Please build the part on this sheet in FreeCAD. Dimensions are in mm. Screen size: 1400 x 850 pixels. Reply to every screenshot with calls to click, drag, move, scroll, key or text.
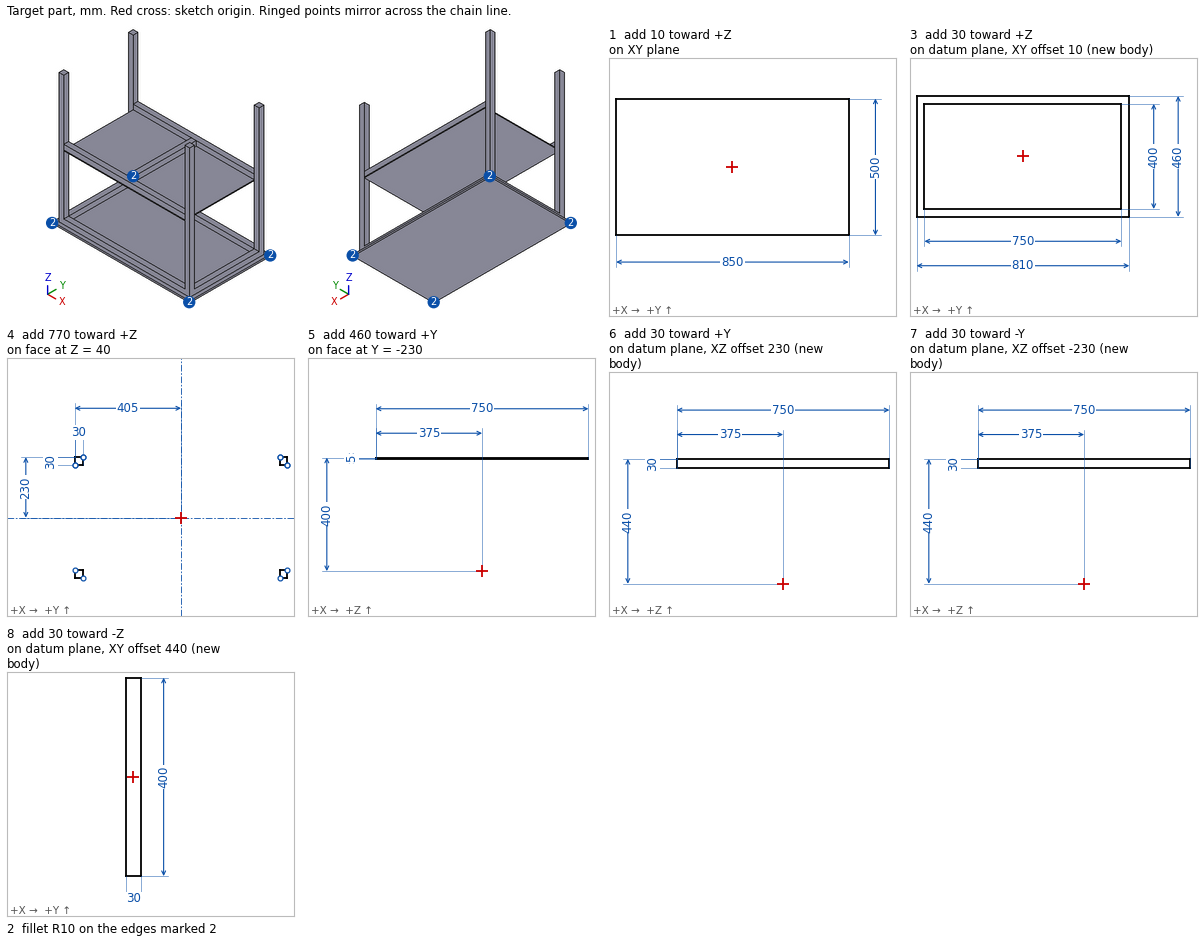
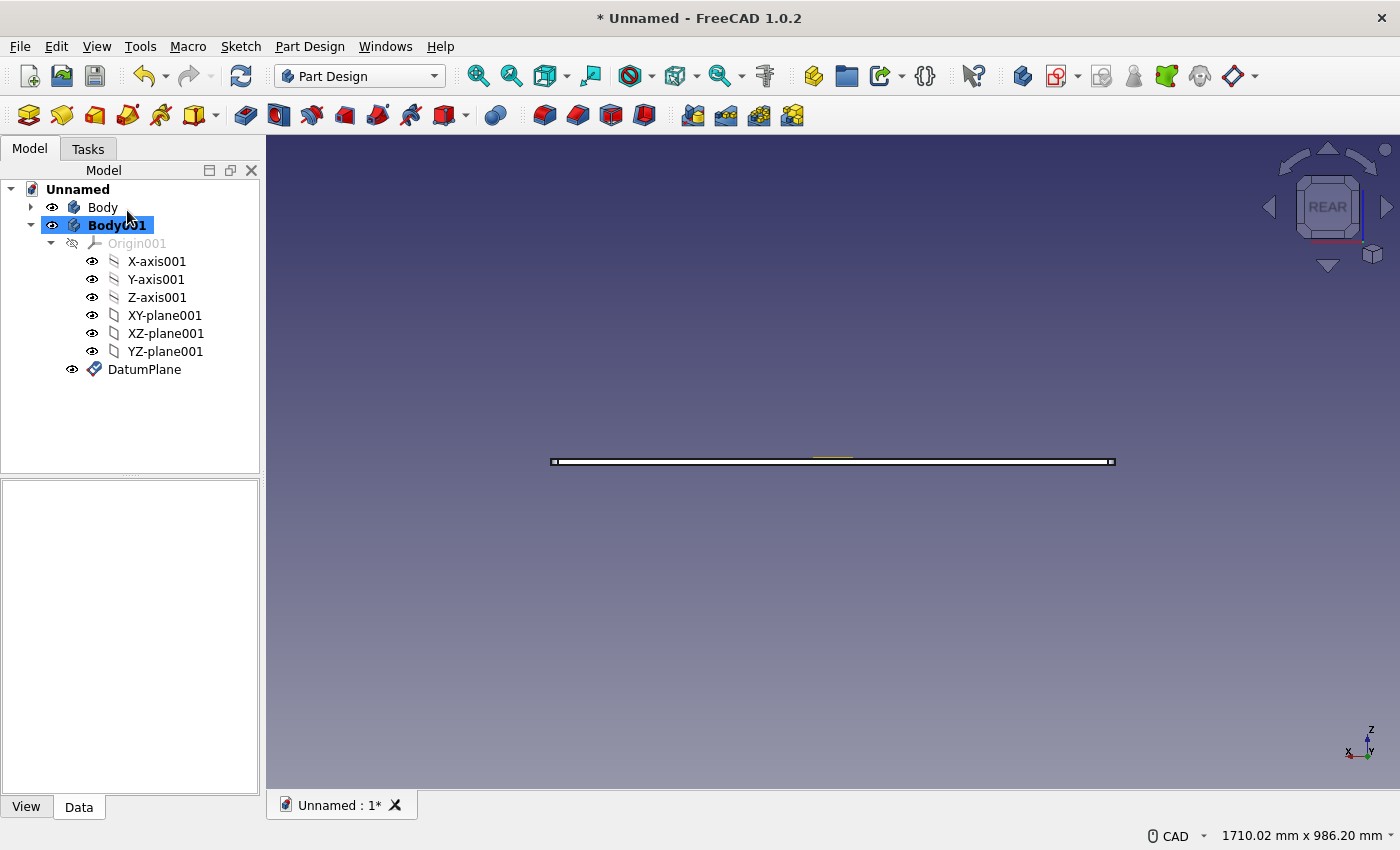
click(117, 369)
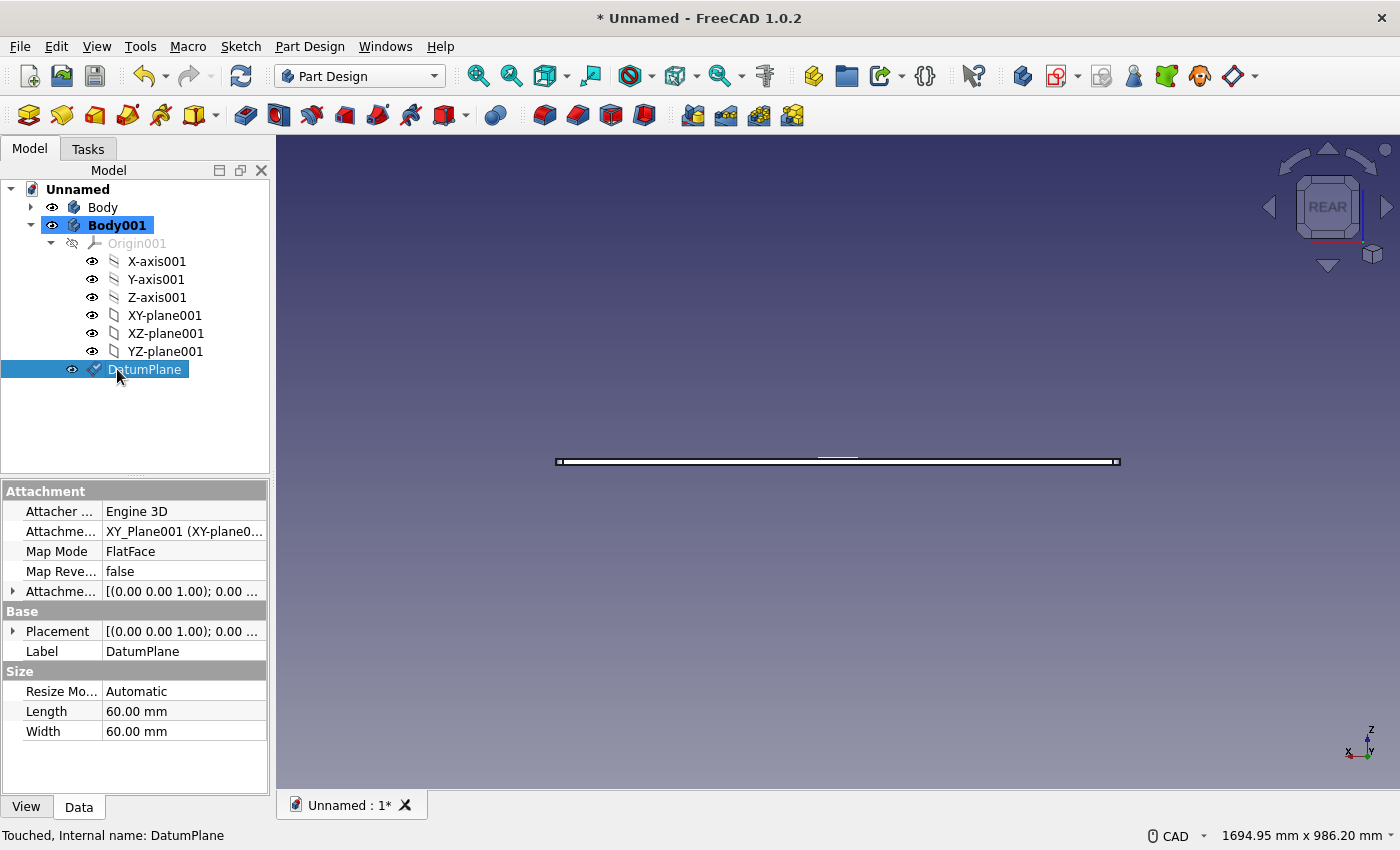
click(1056, 76)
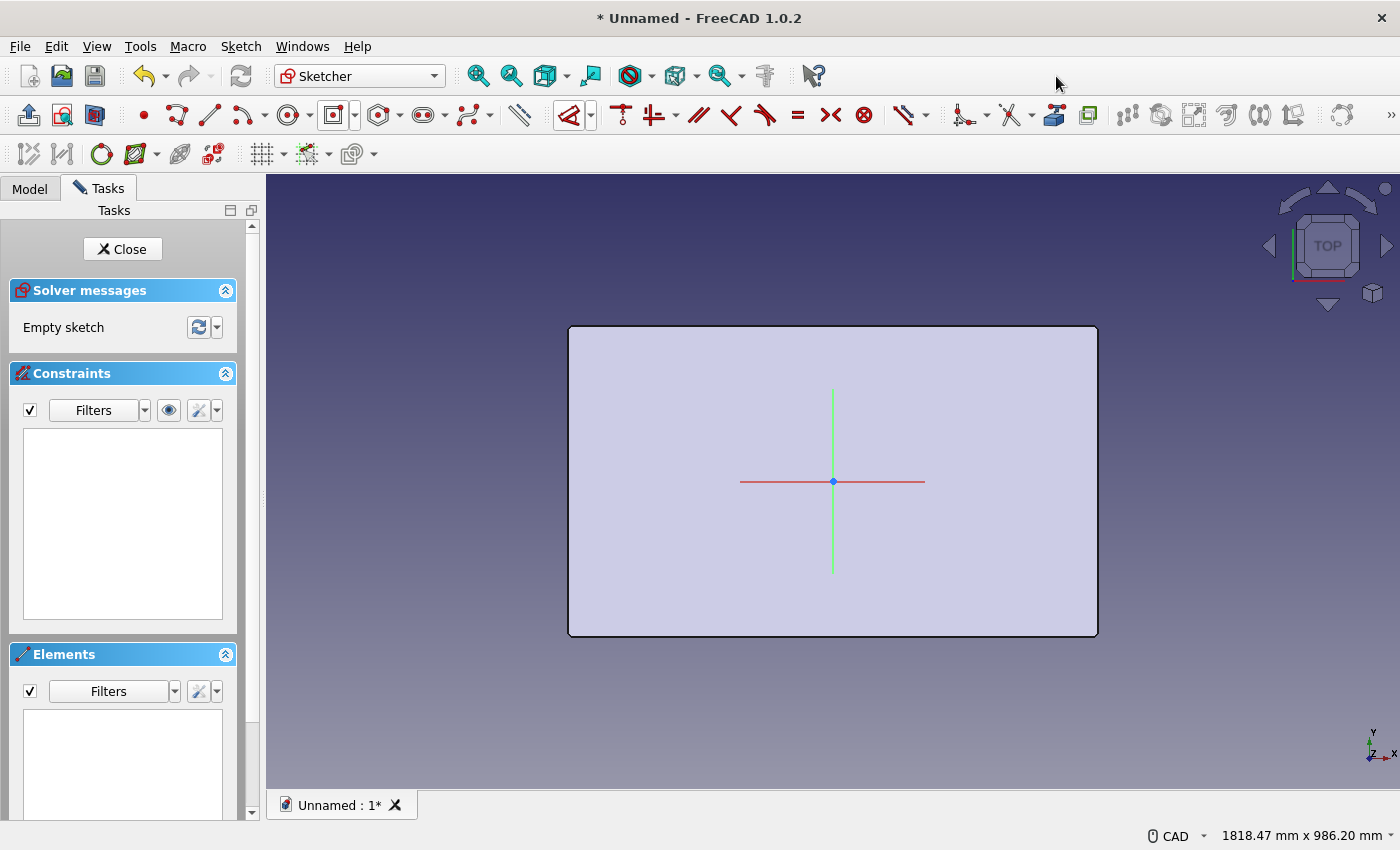
click(332, 116)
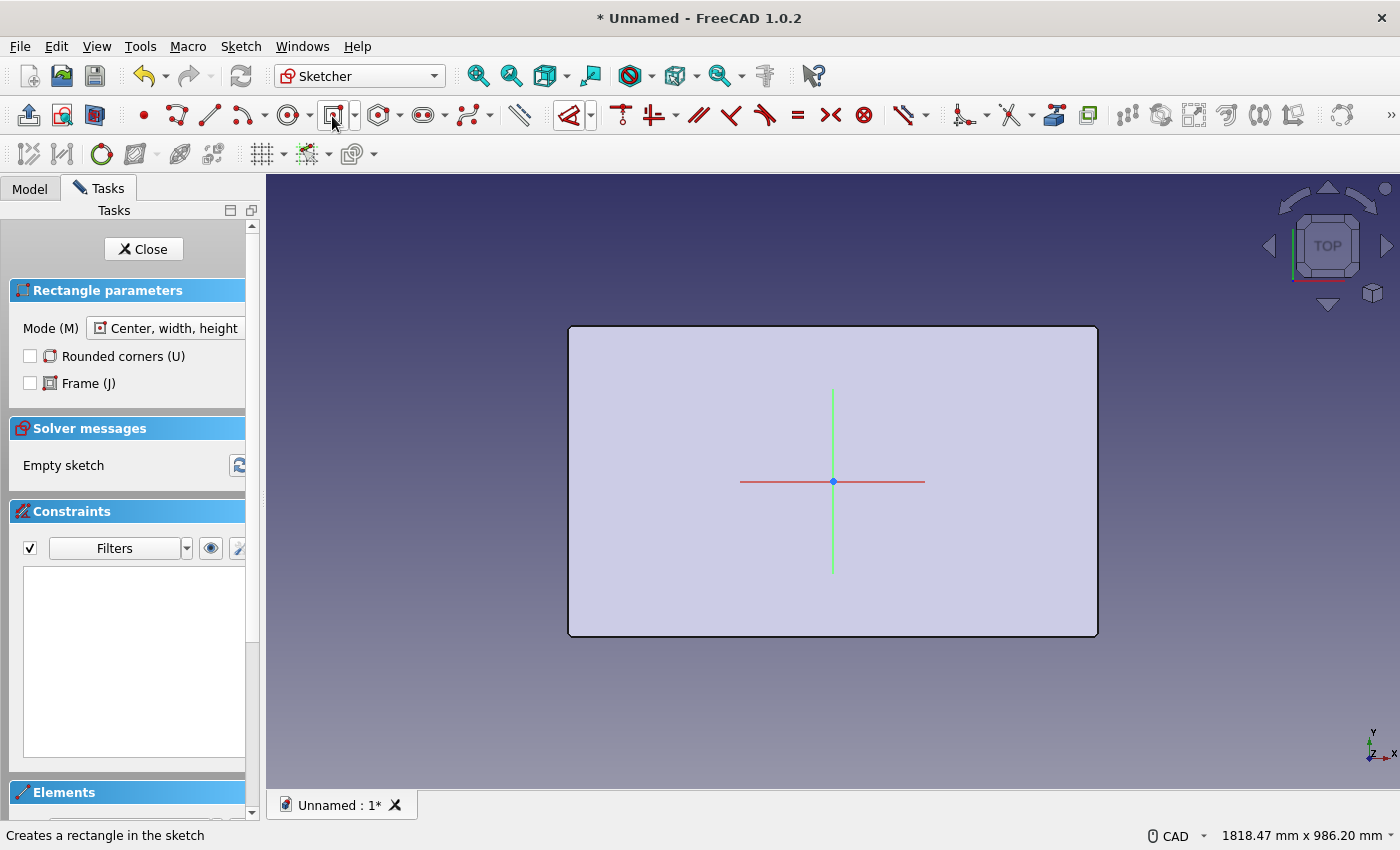
click(833, 482)
click(1086, 338)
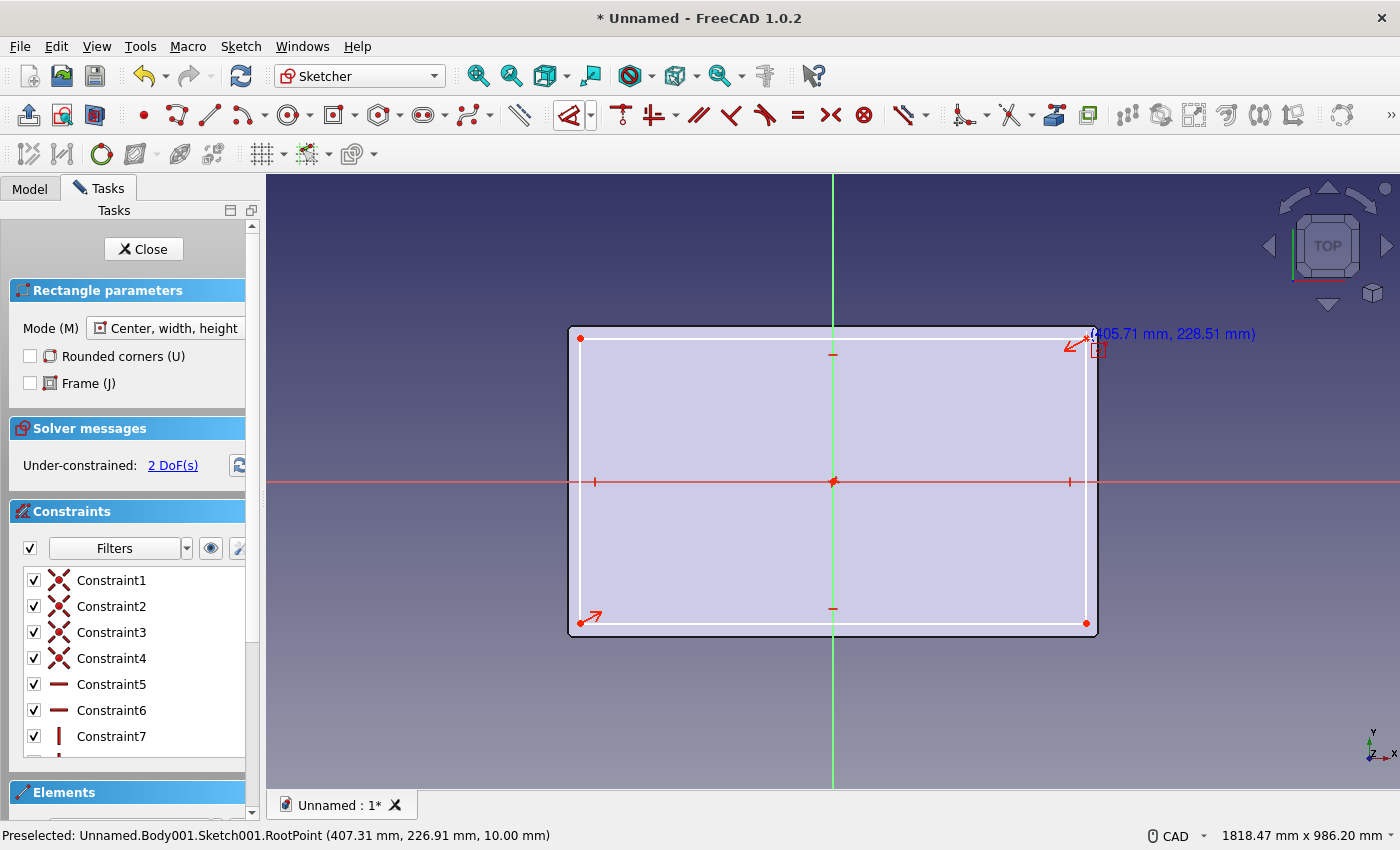
click(833, 482)
click(1067, 357)
key(Escape)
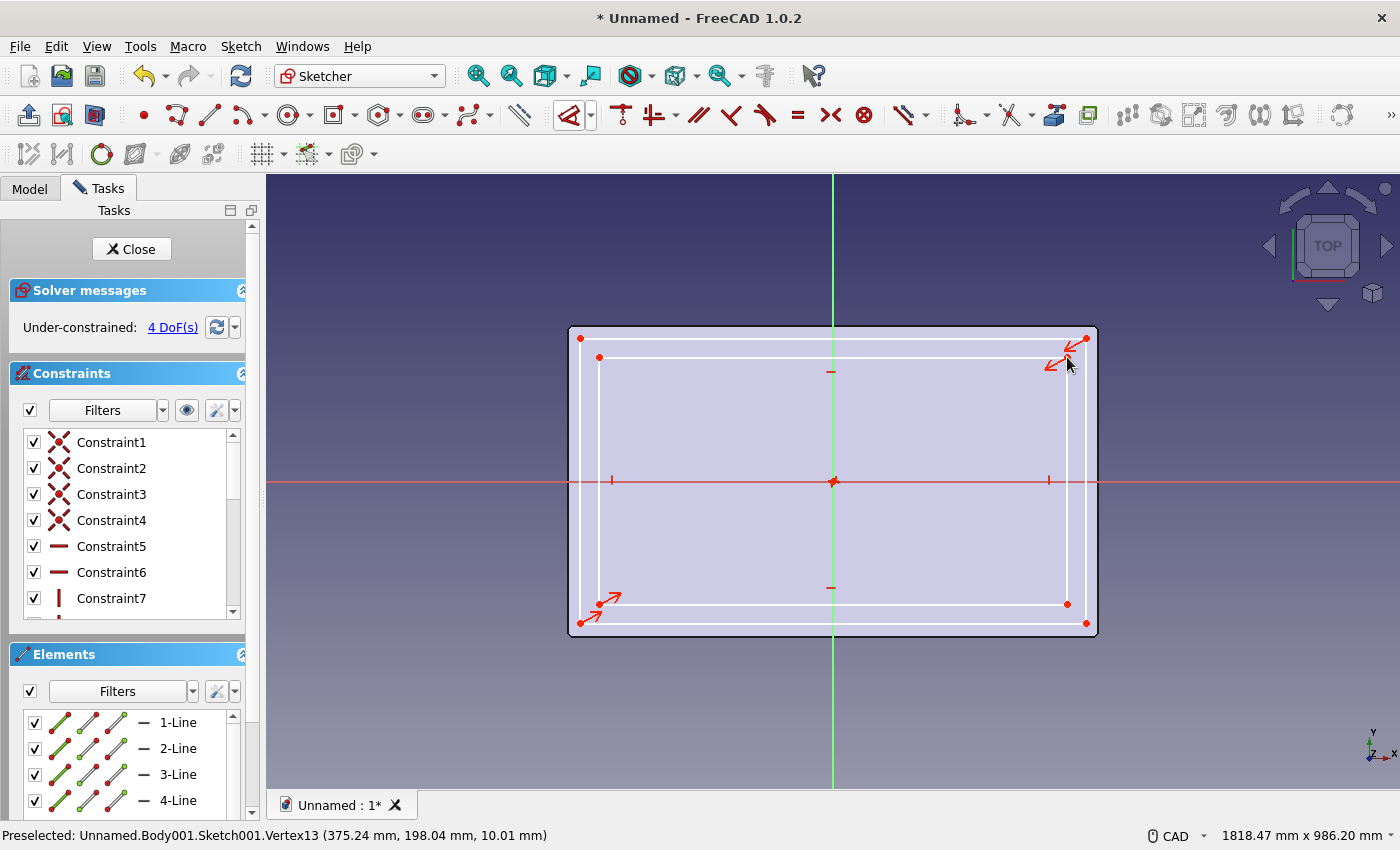
click(732, 624)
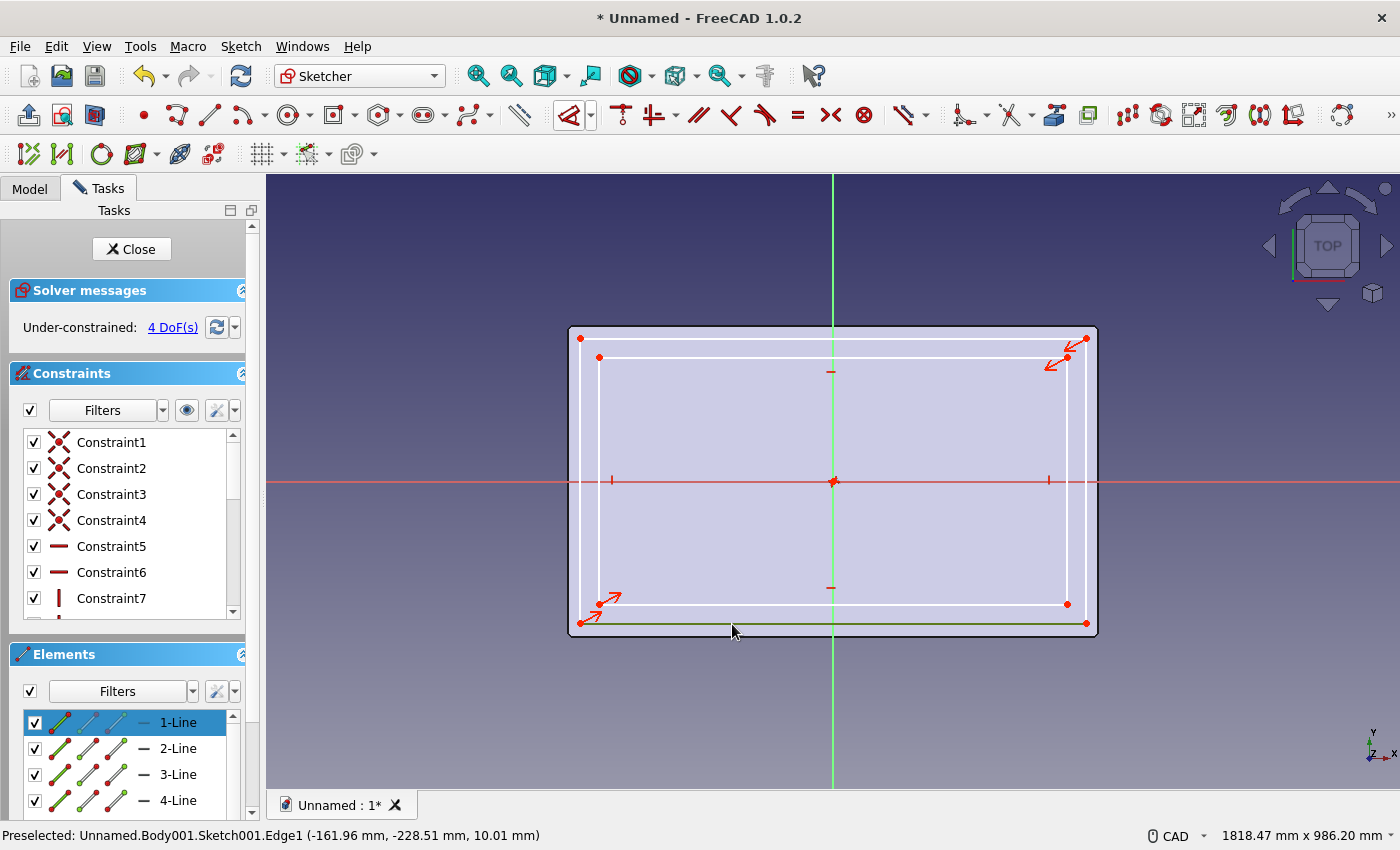
click(590, 116)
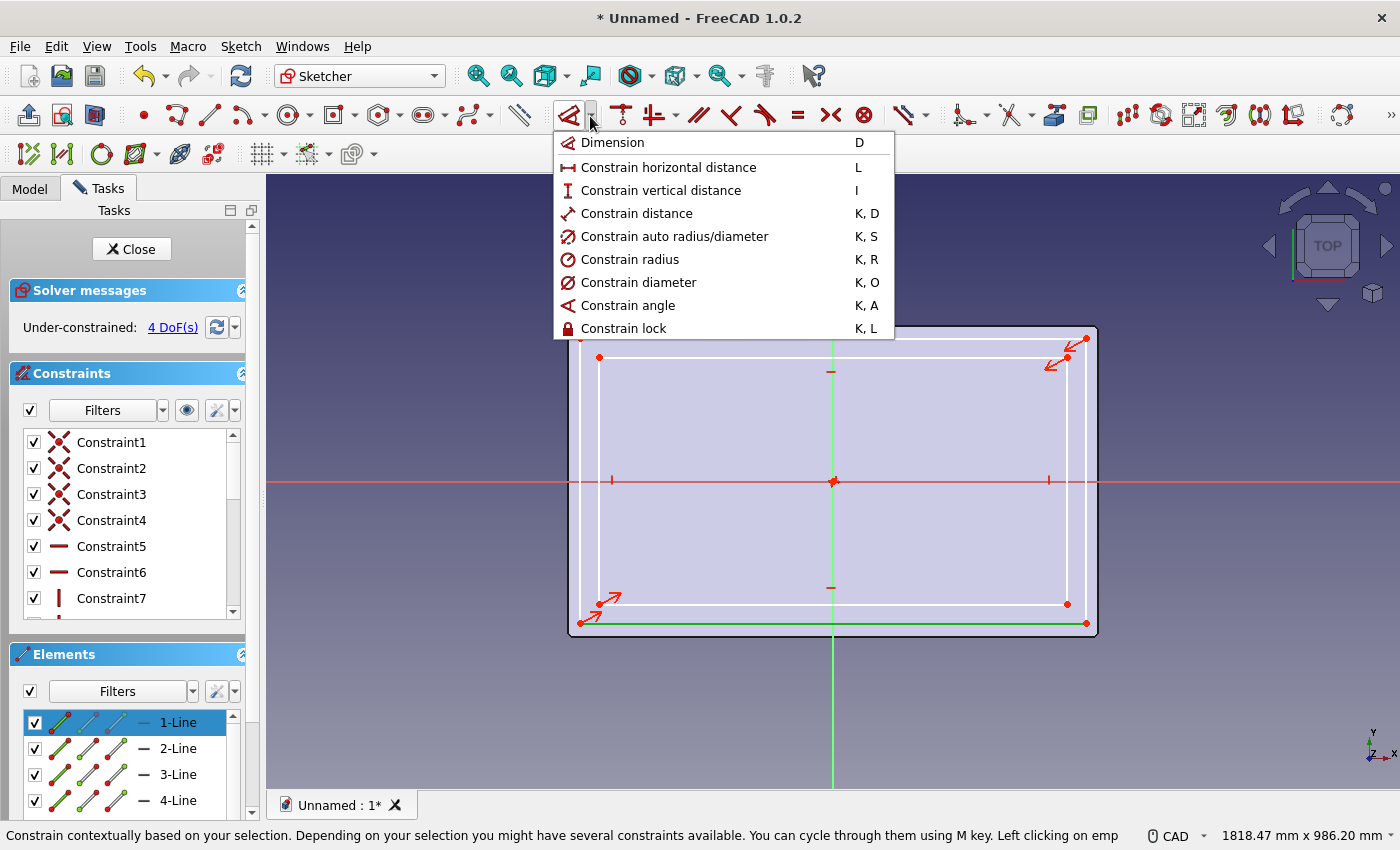
click(724, 168)